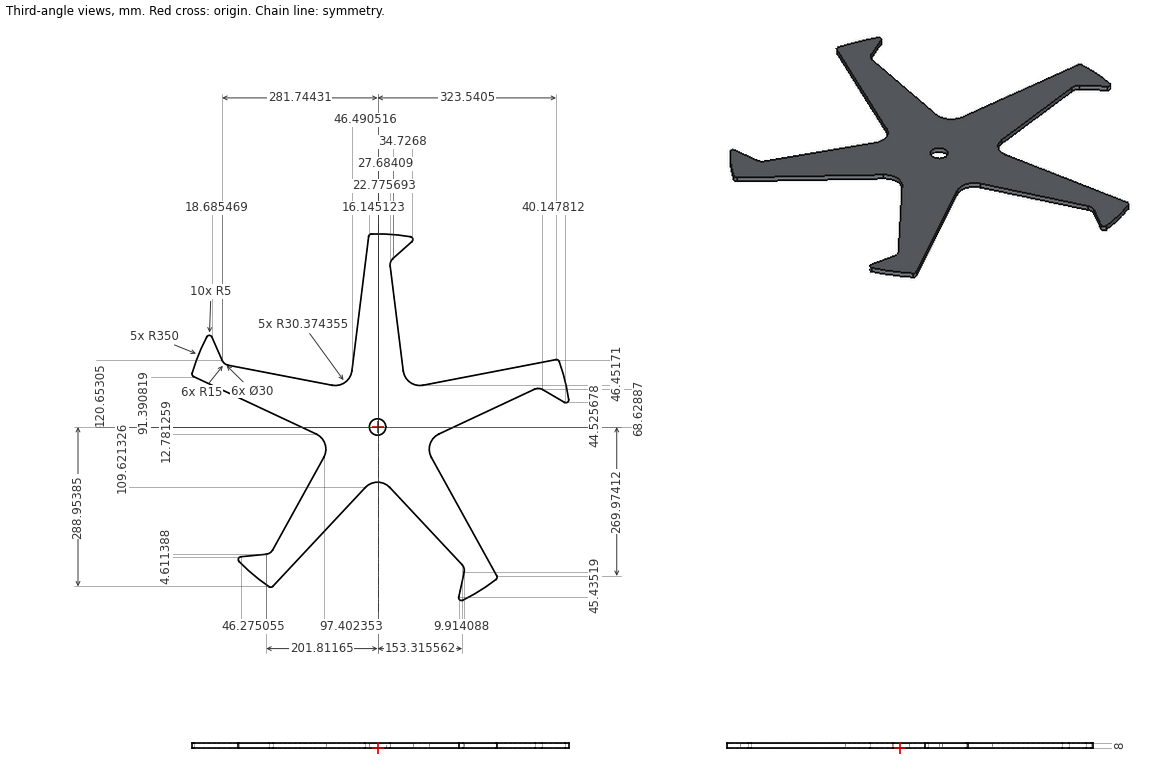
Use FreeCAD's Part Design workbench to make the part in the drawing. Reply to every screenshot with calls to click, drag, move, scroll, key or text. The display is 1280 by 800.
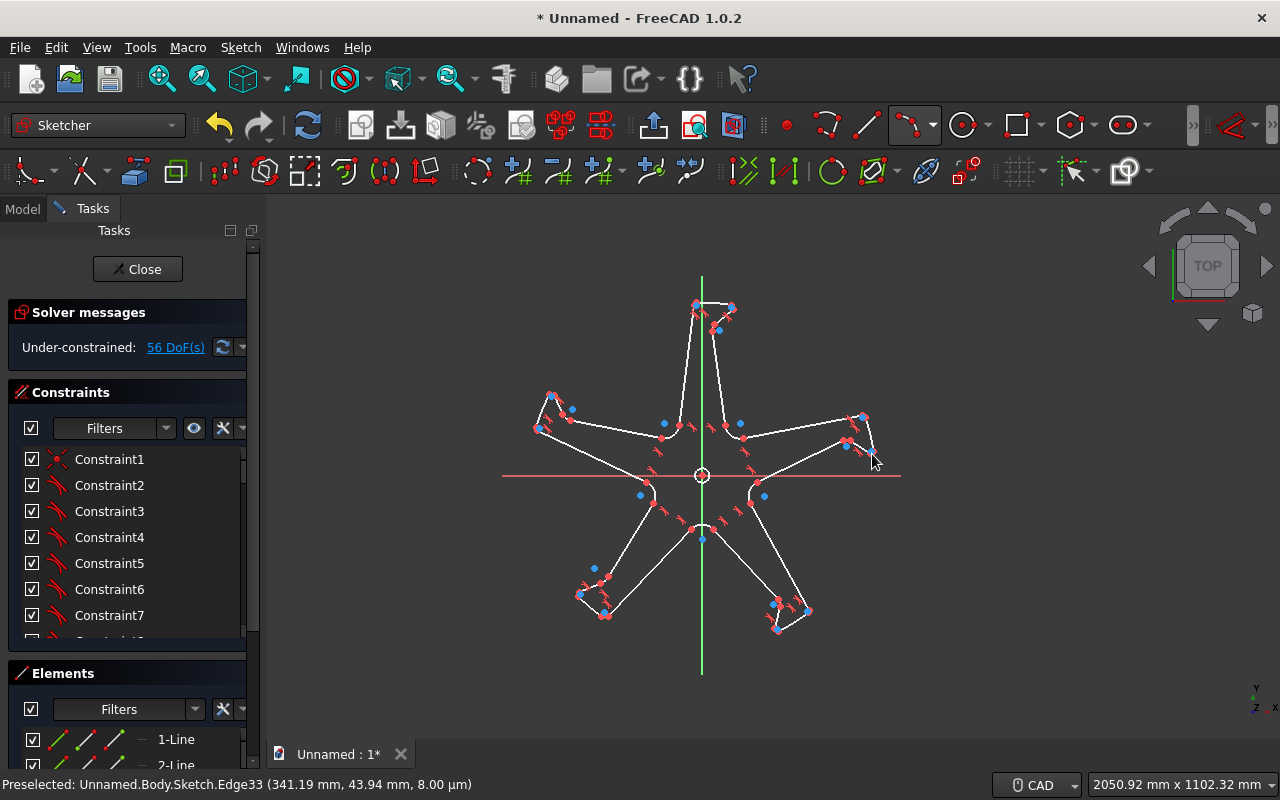
scroll(865, 416, up, 14)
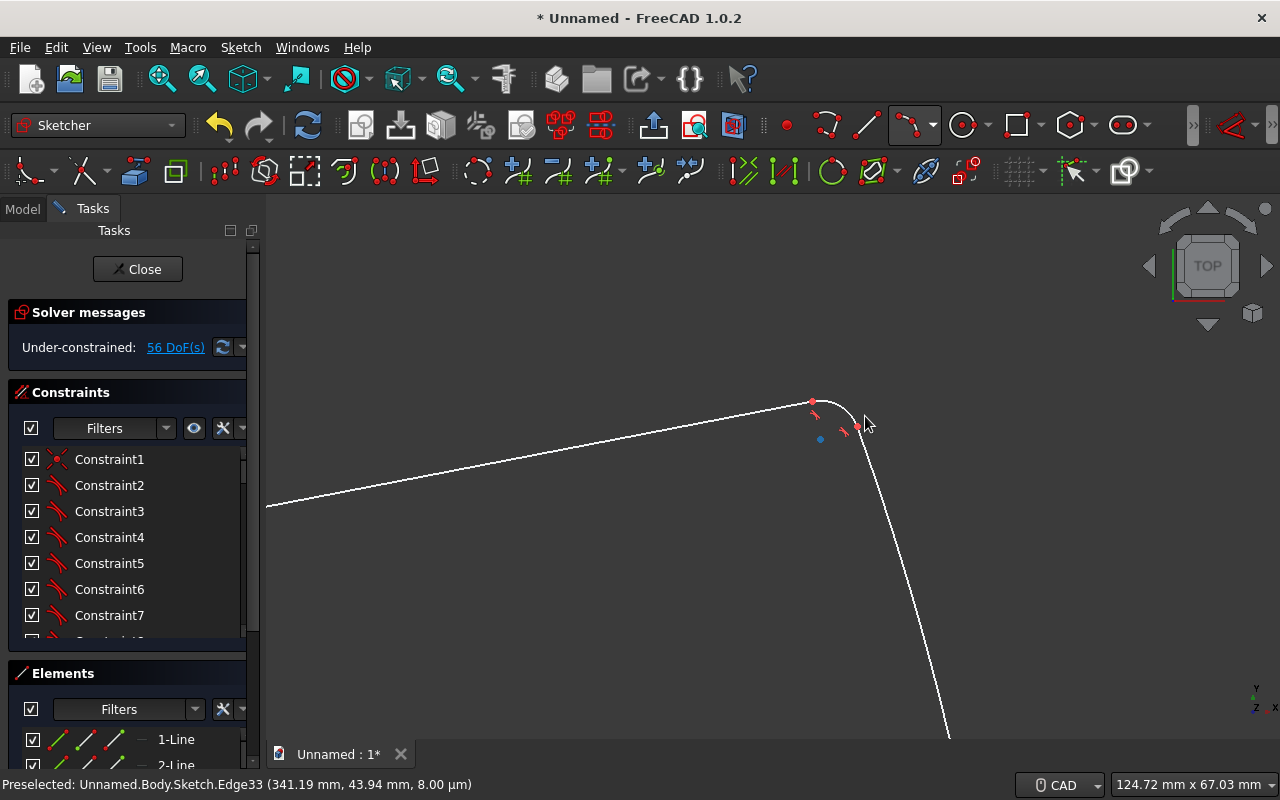
click(848, 413)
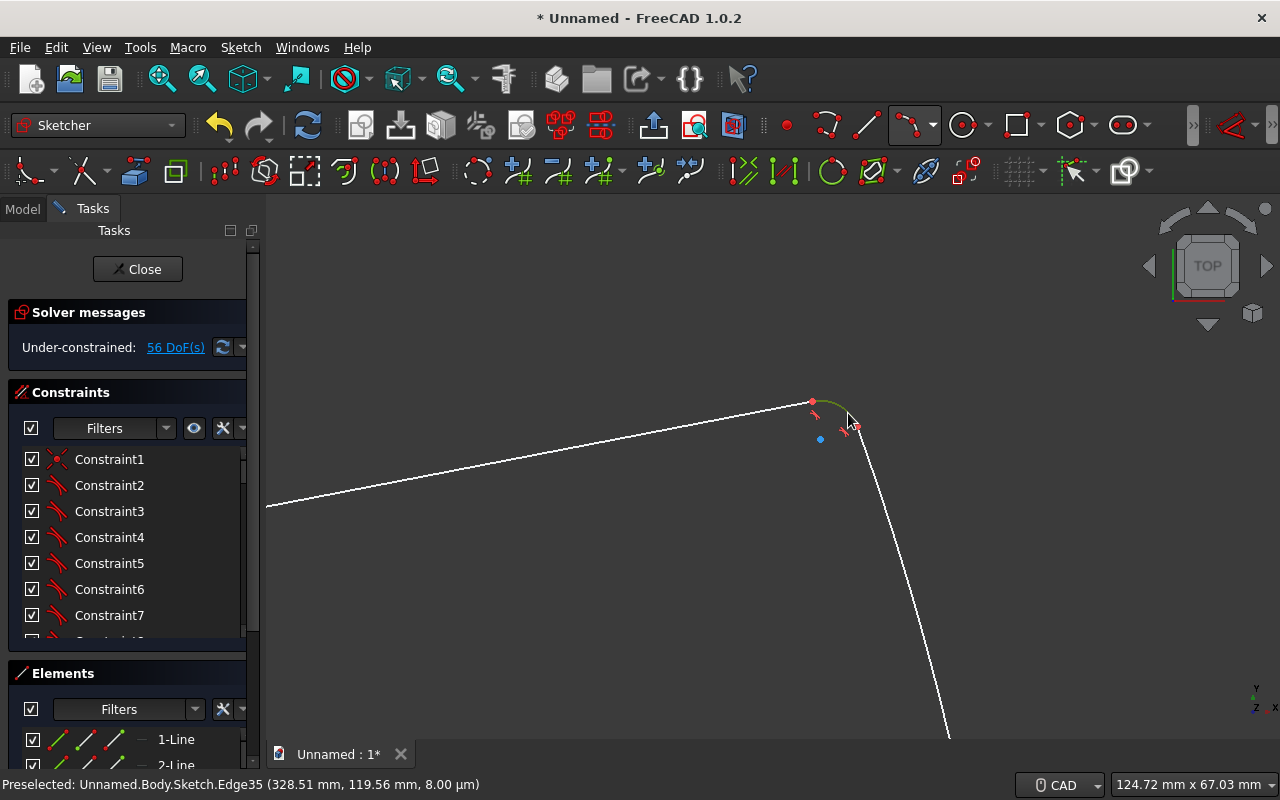
scroll(865, 416, down, 14)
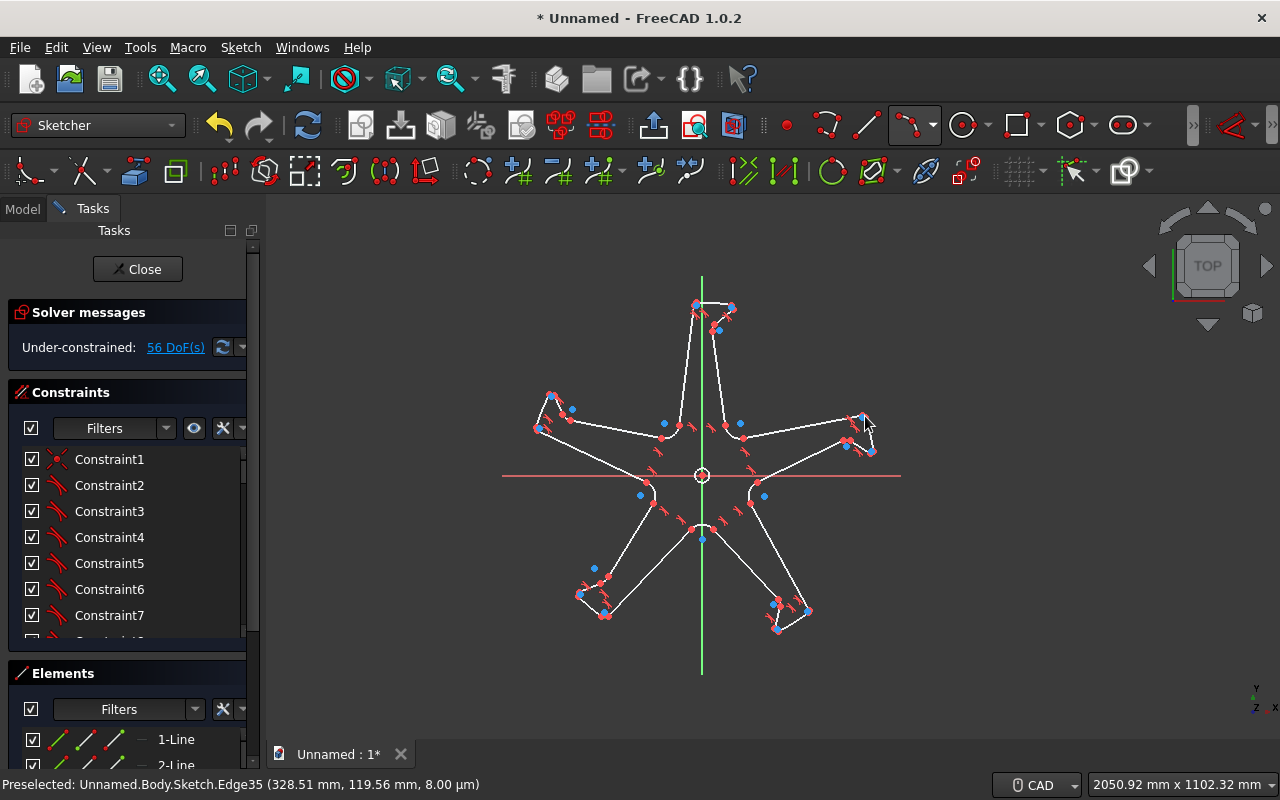
scroll(734, 308, up, 11)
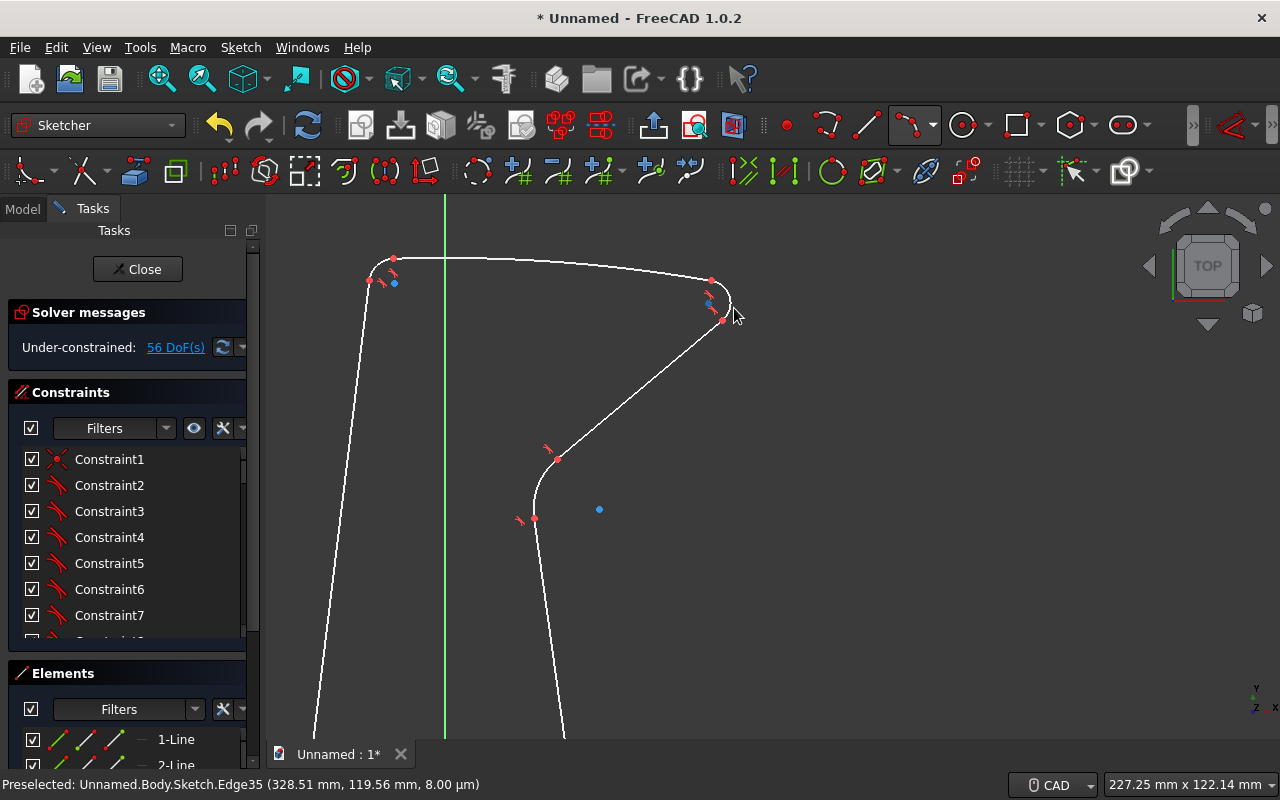
click(730, 307)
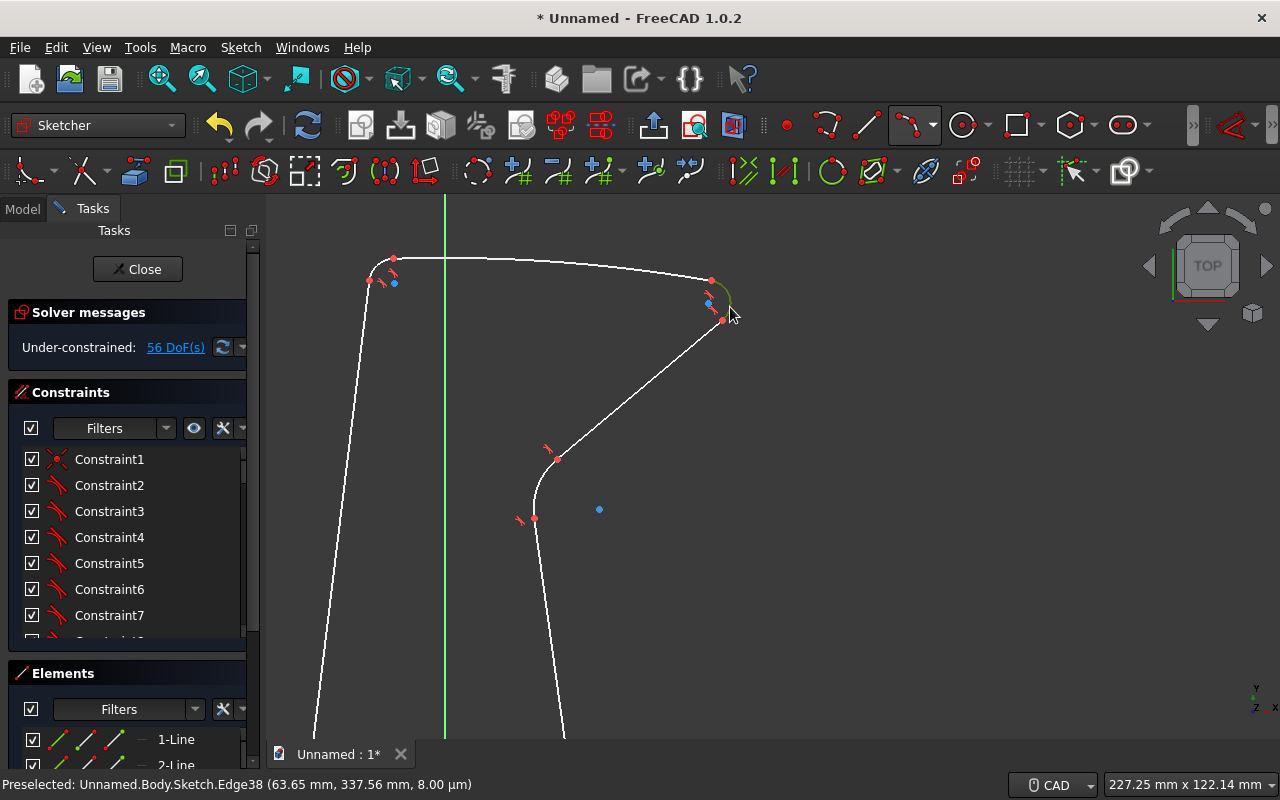
scroll(383, 261, up, 2)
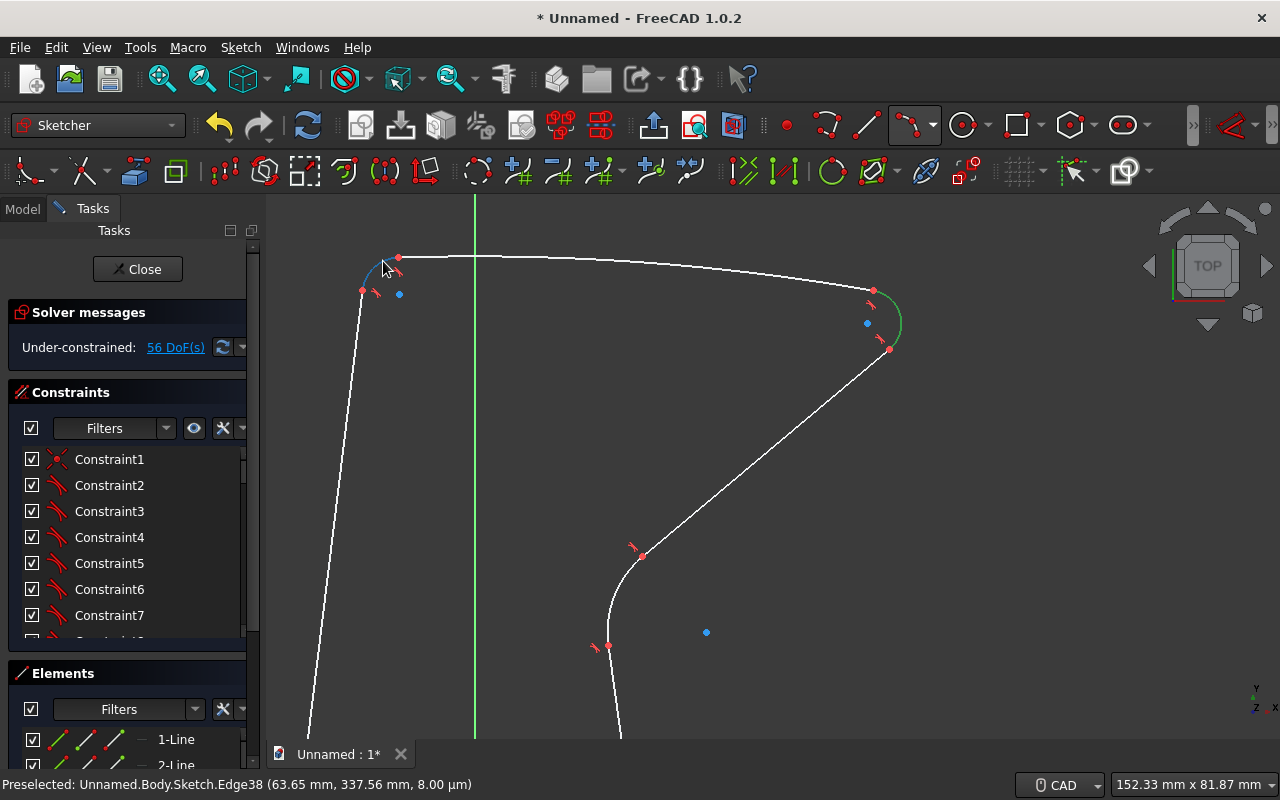
click(383, 261)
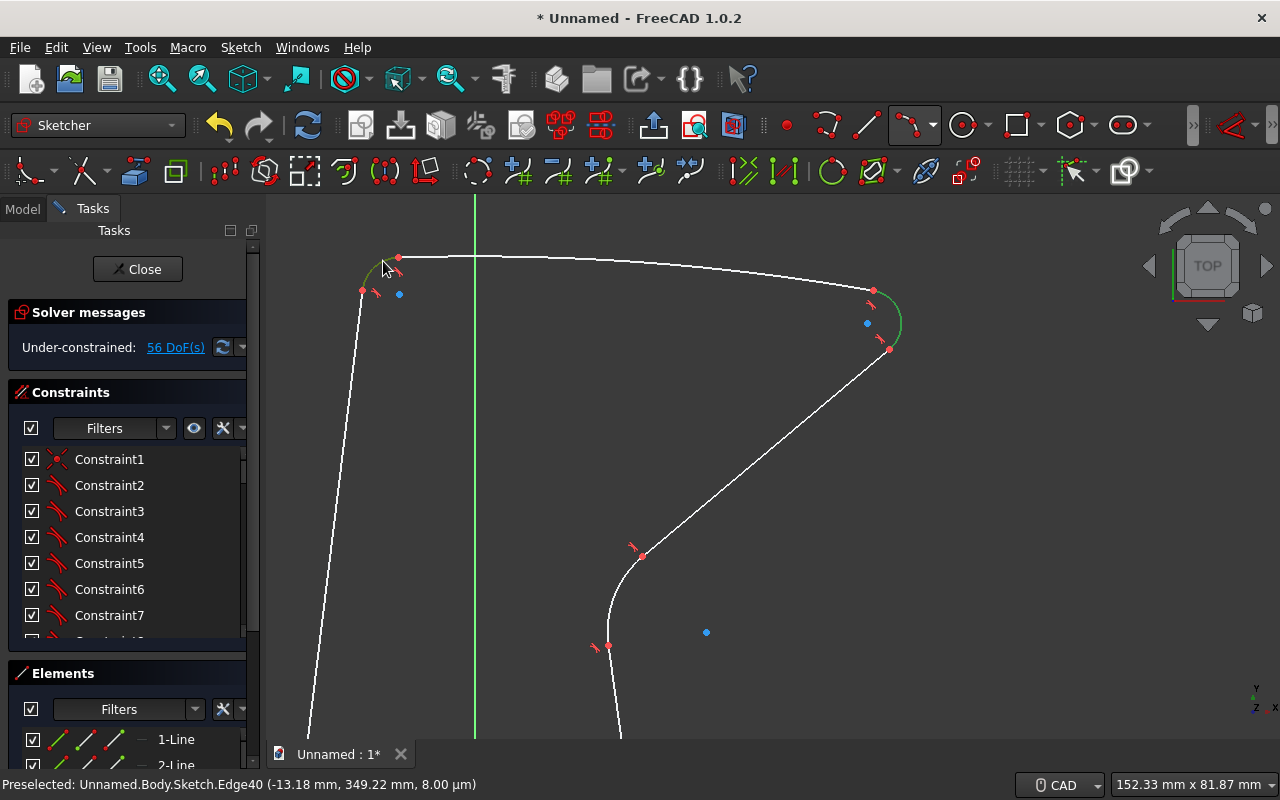
key(e)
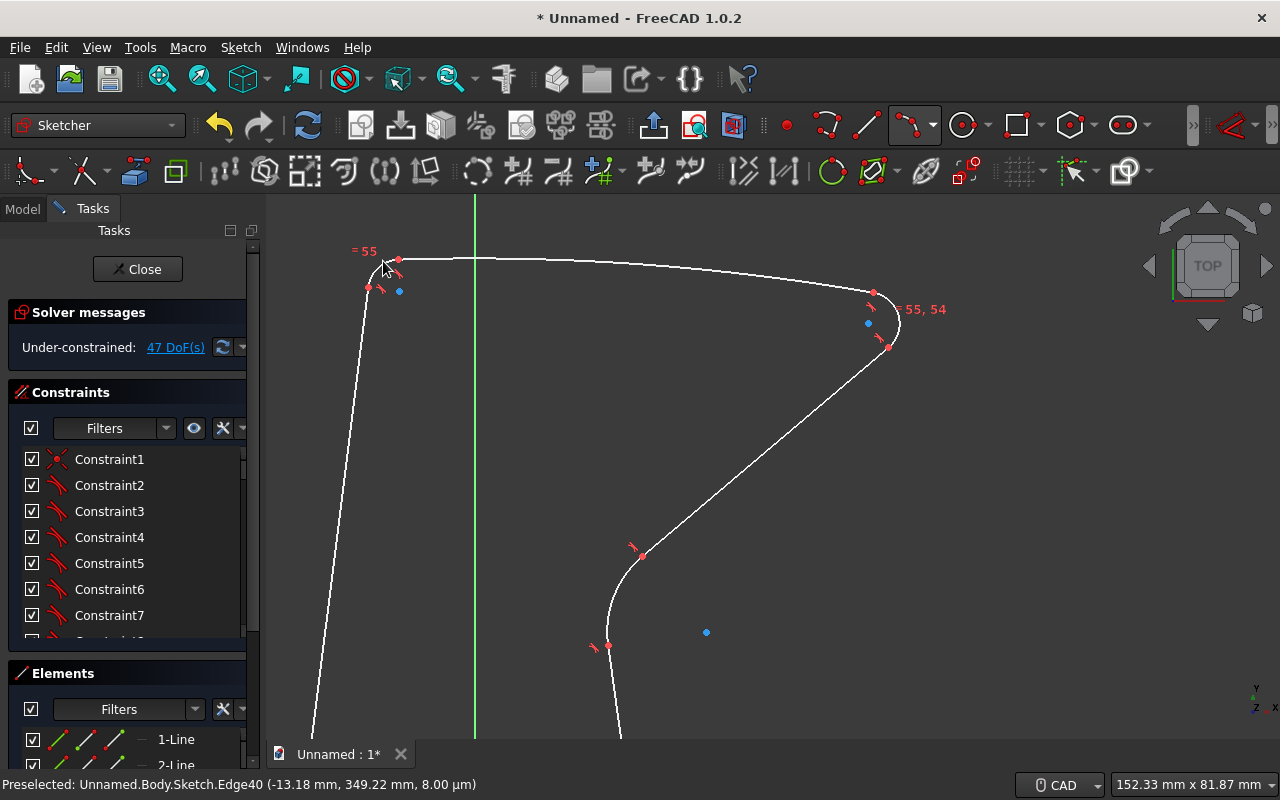
scroll(720, 306, down, 13)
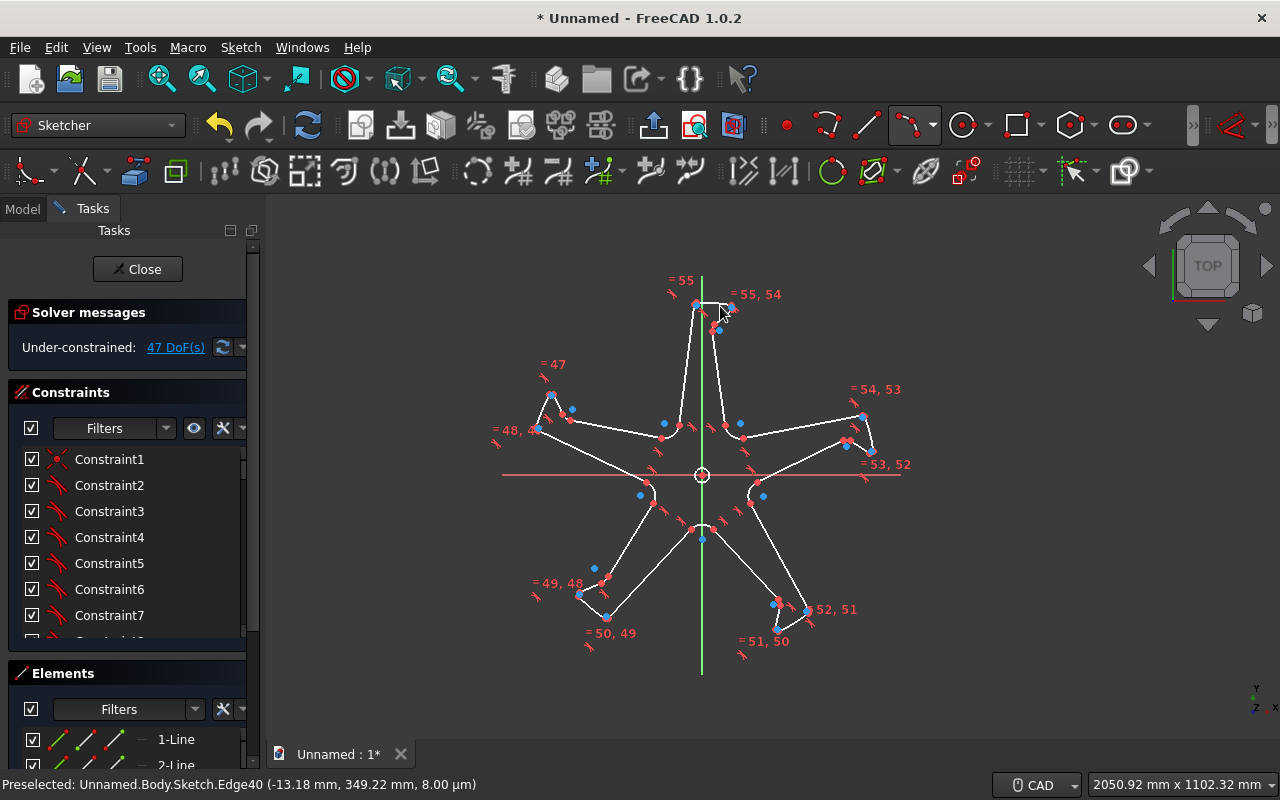
scroll(669, 438, up, 4)